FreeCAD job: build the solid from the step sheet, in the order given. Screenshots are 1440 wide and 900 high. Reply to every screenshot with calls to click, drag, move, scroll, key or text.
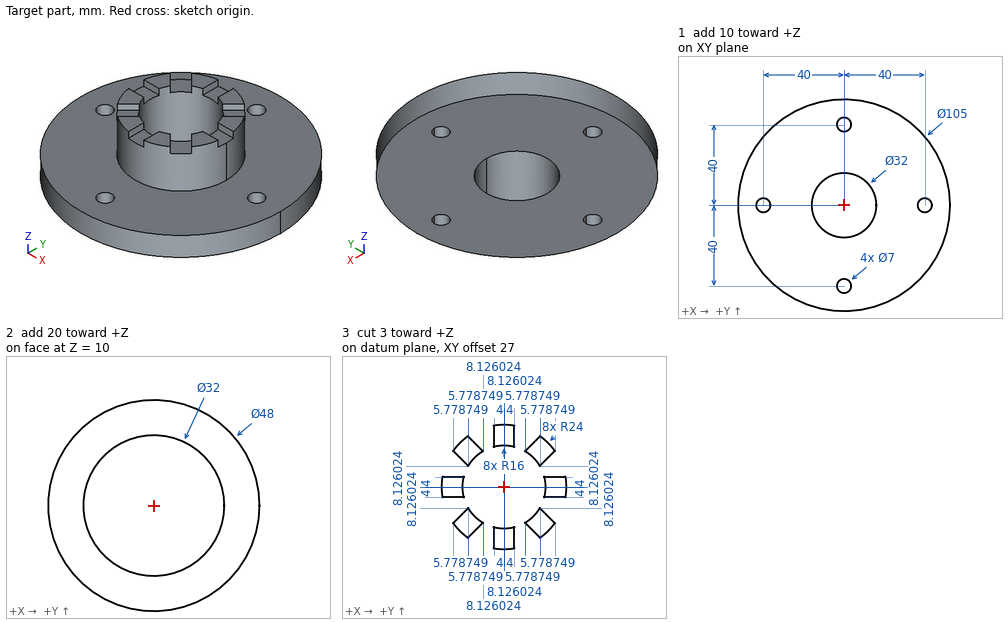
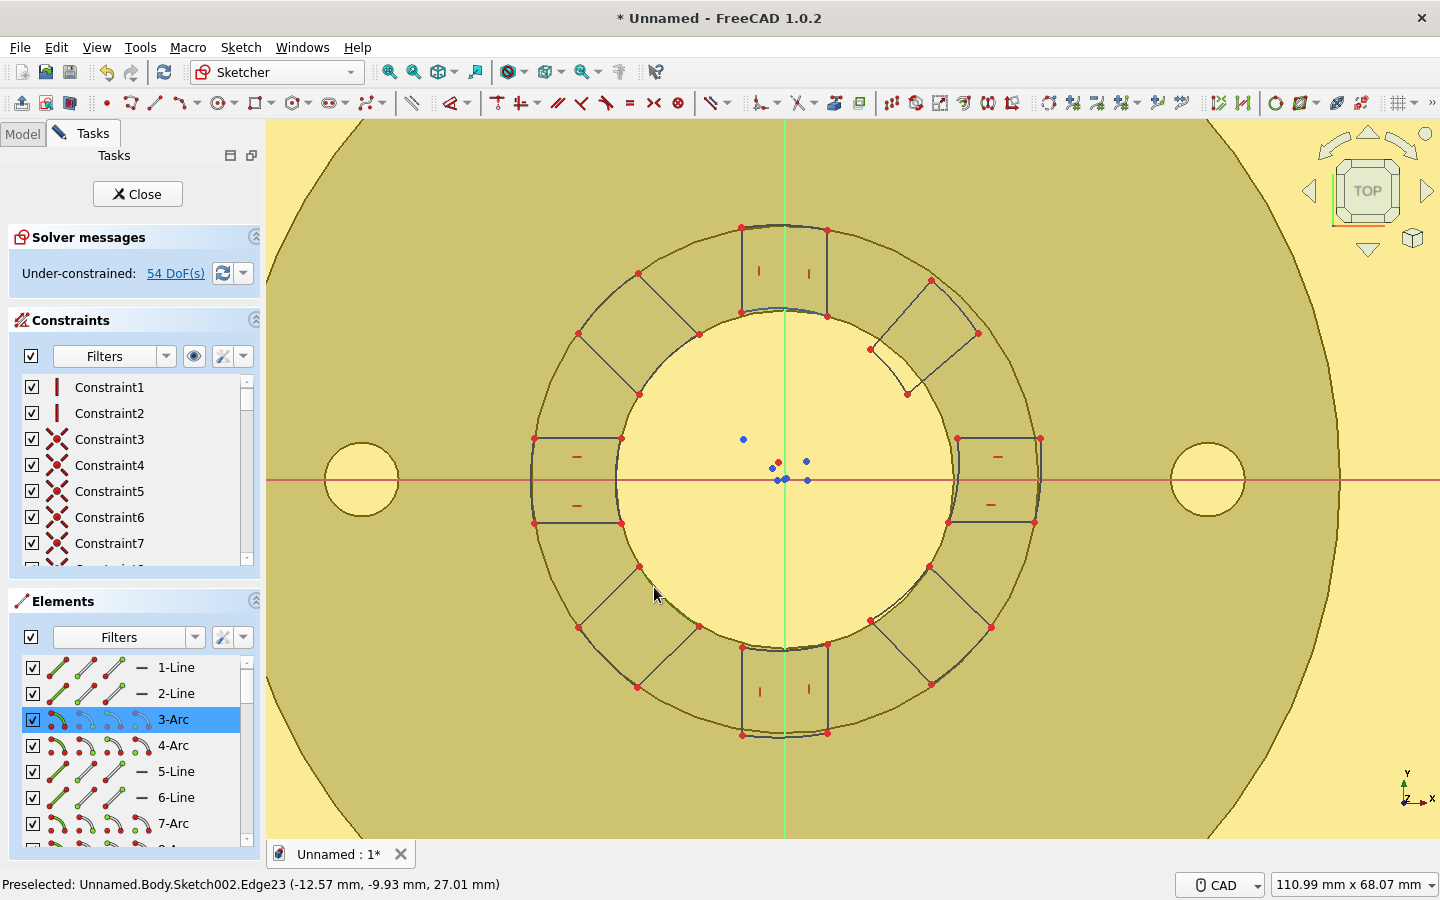
click(498, 104)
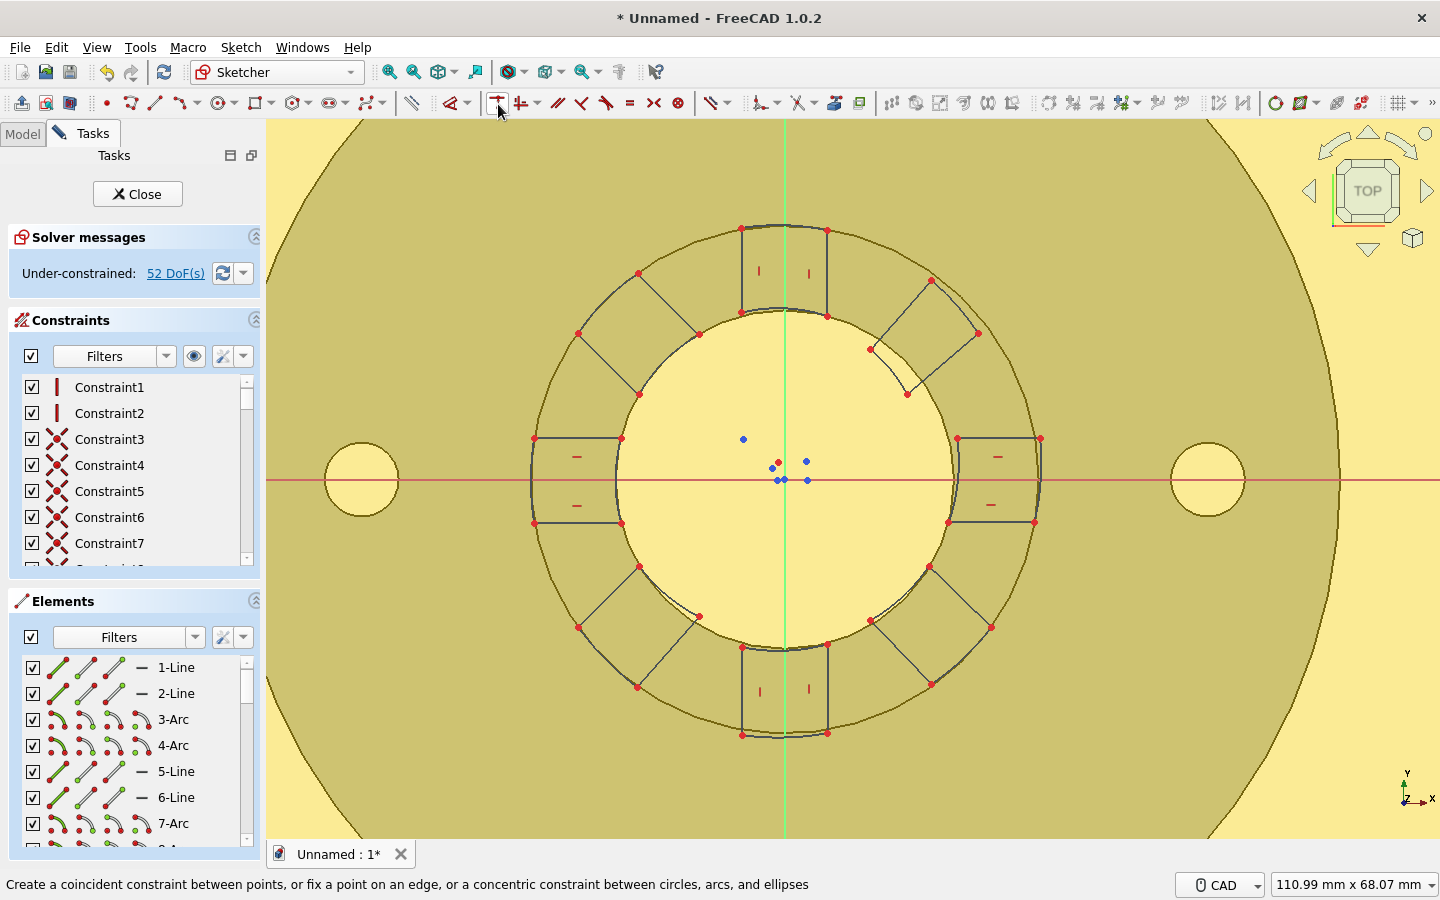
click(802, 310)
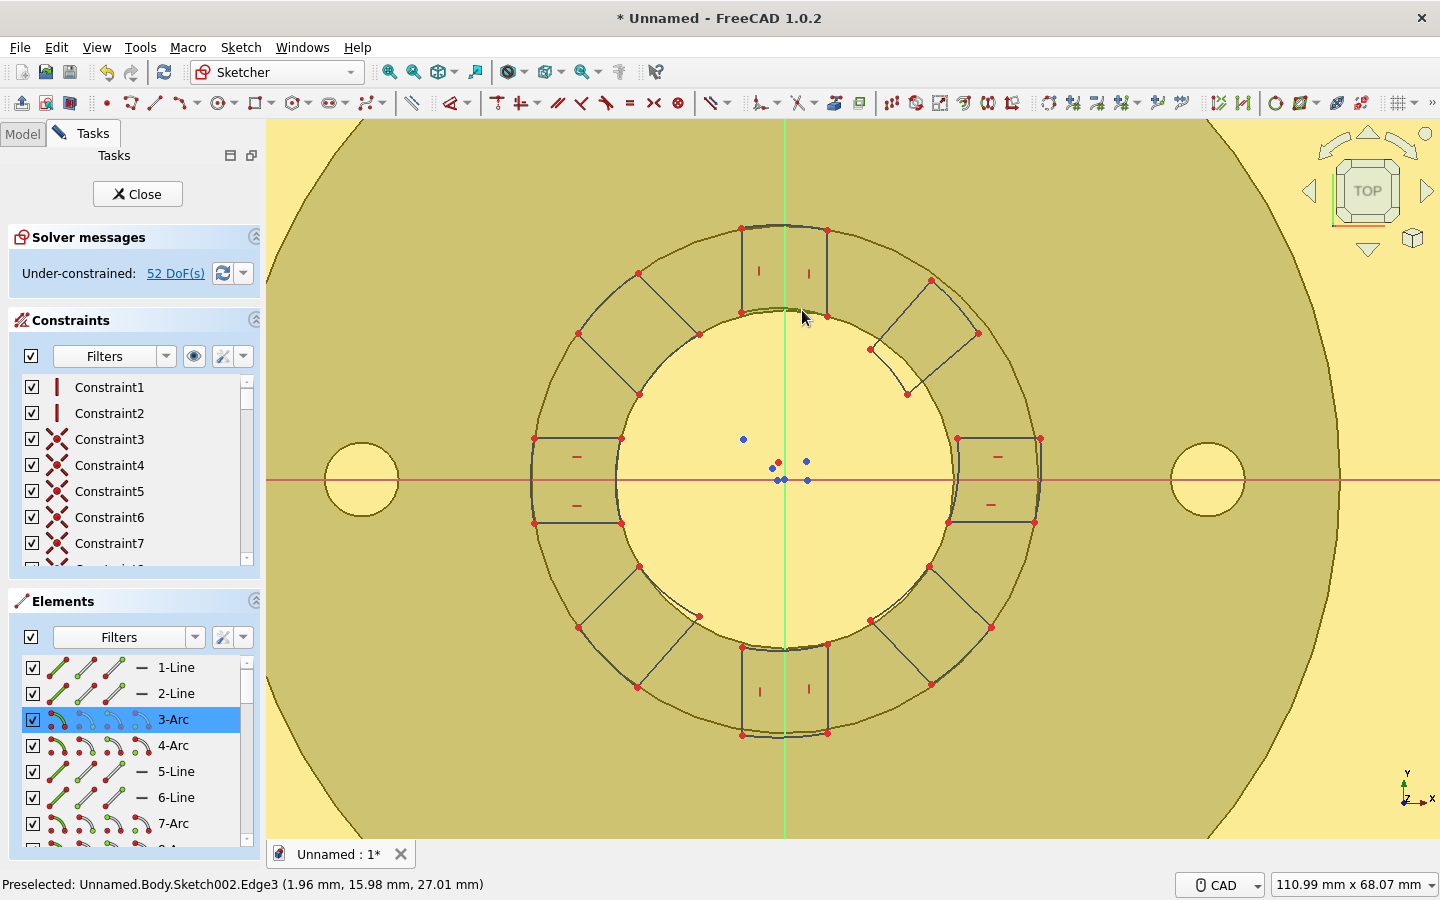
click(594, 647)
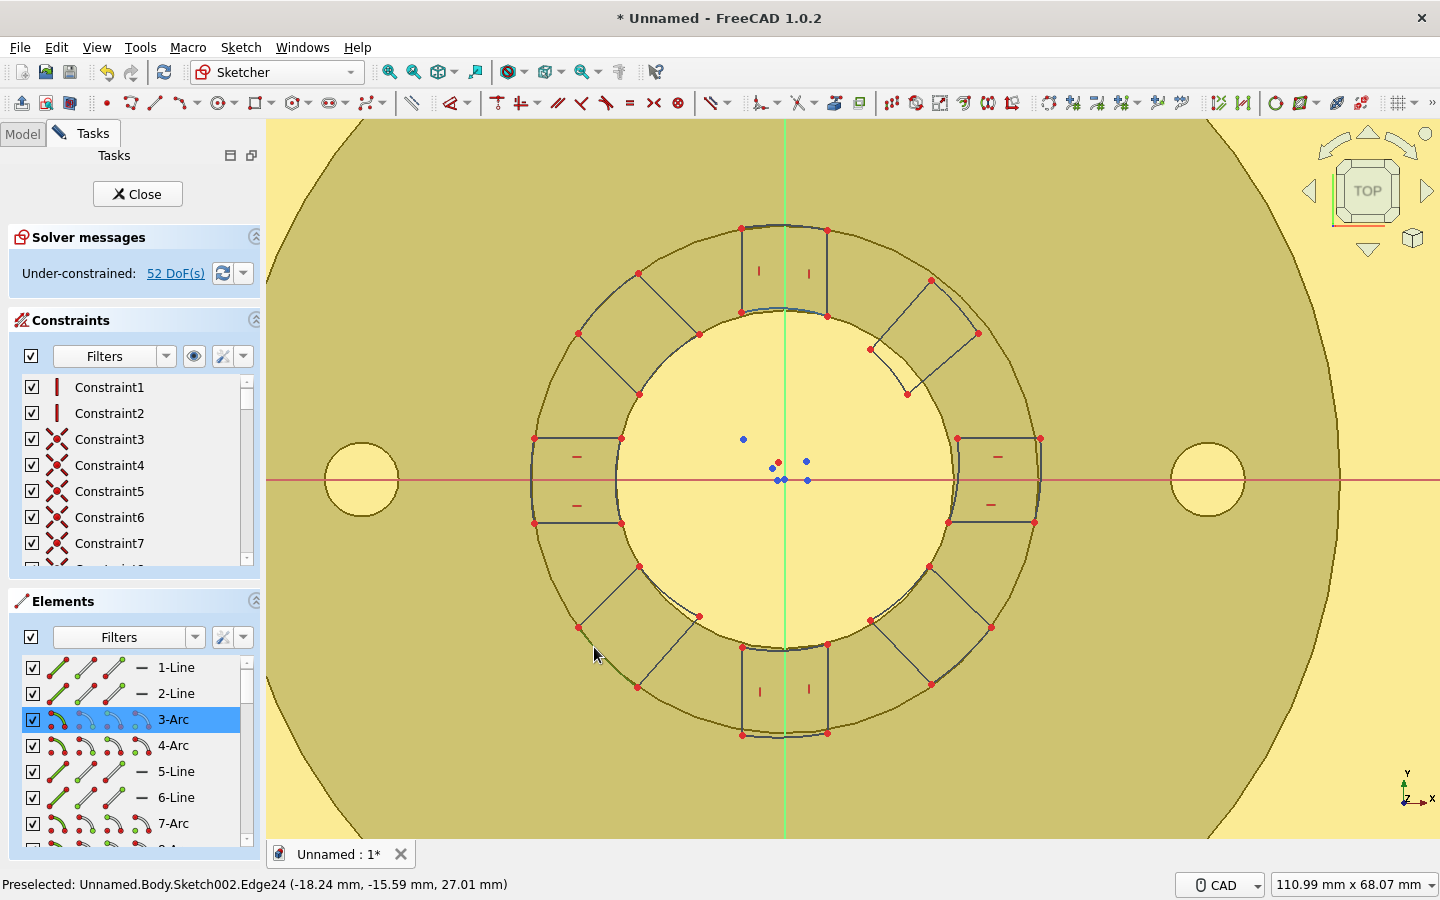
click(498, 104)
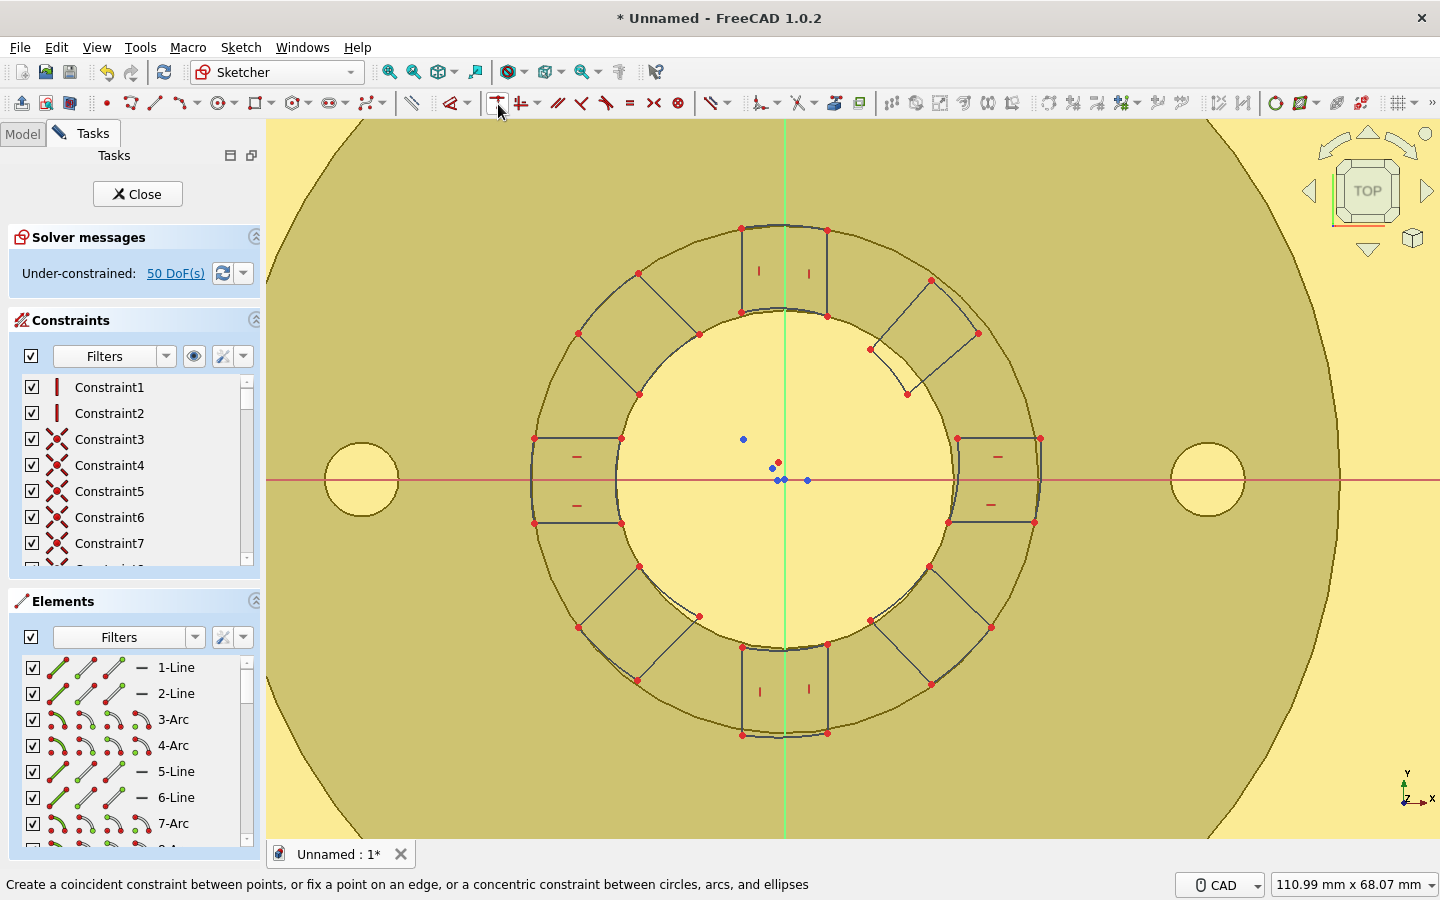
click(802, 310)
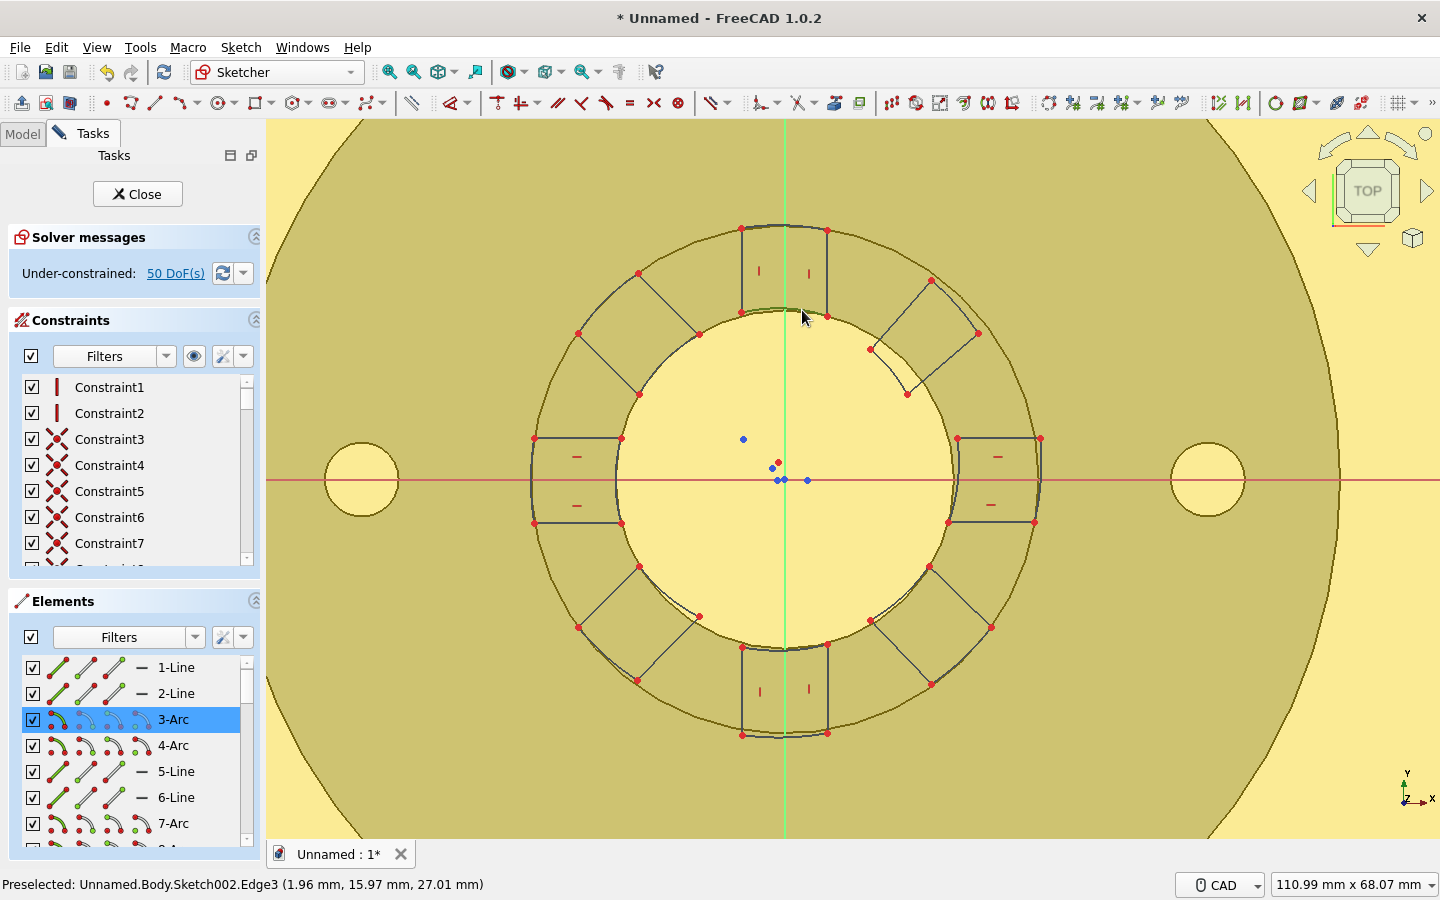
click(617, 464)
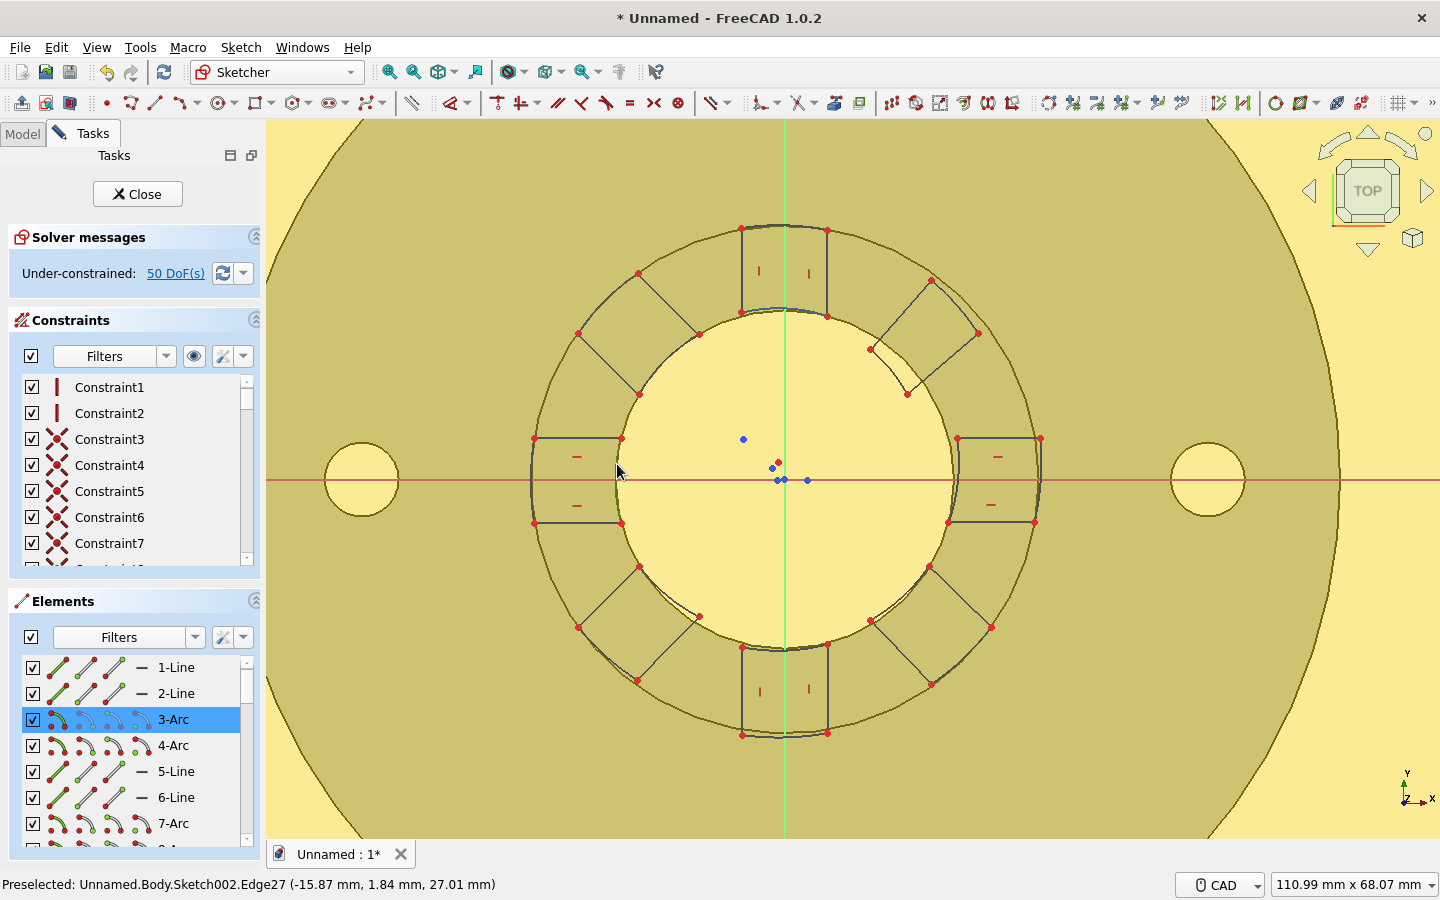
click(498, 104)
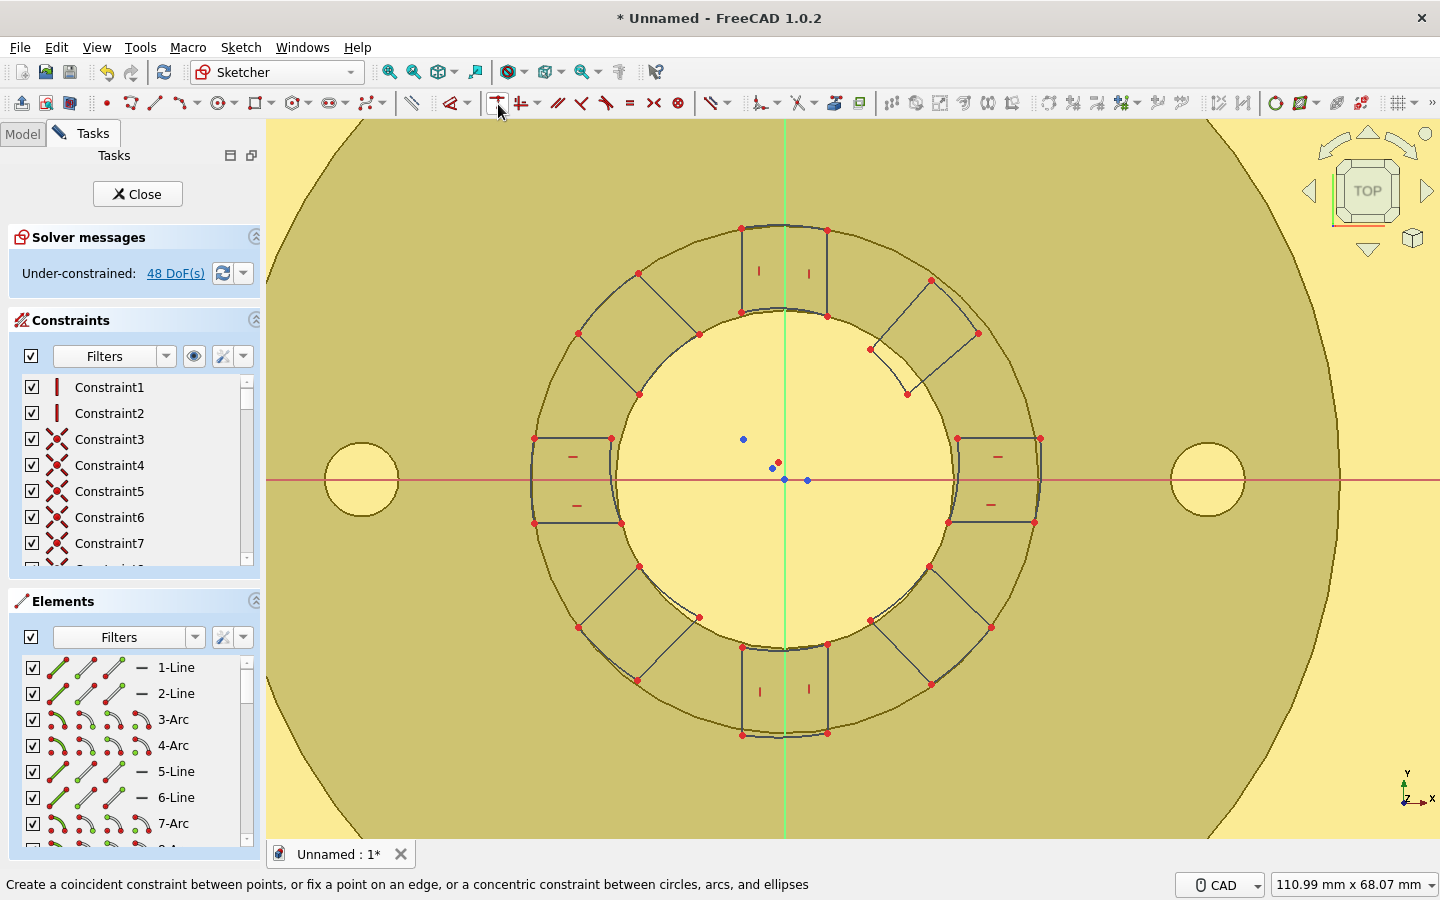
click(802, 310)